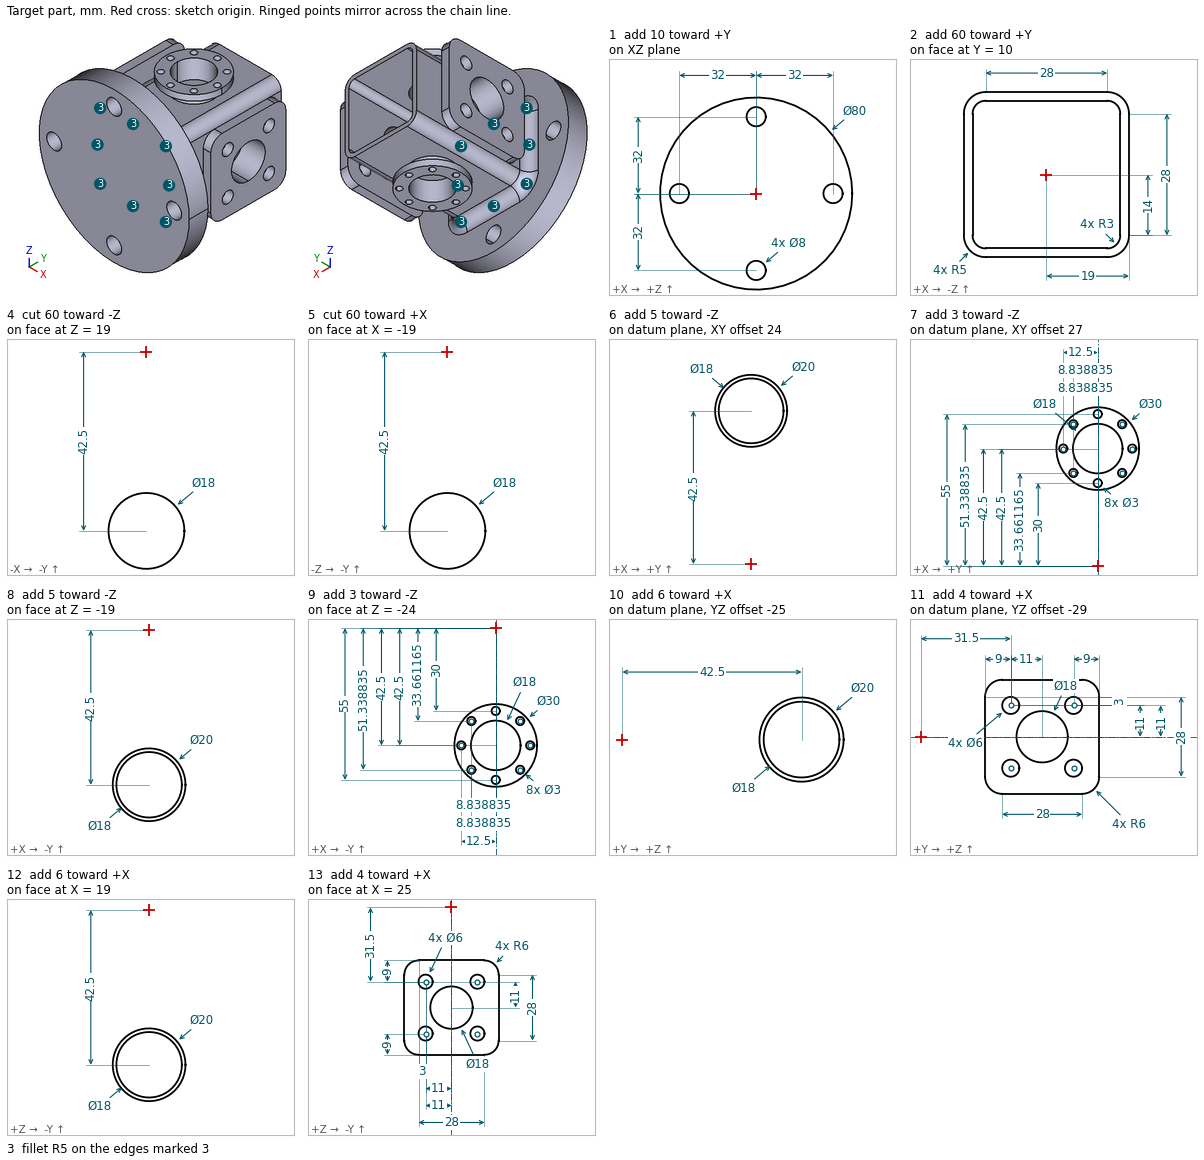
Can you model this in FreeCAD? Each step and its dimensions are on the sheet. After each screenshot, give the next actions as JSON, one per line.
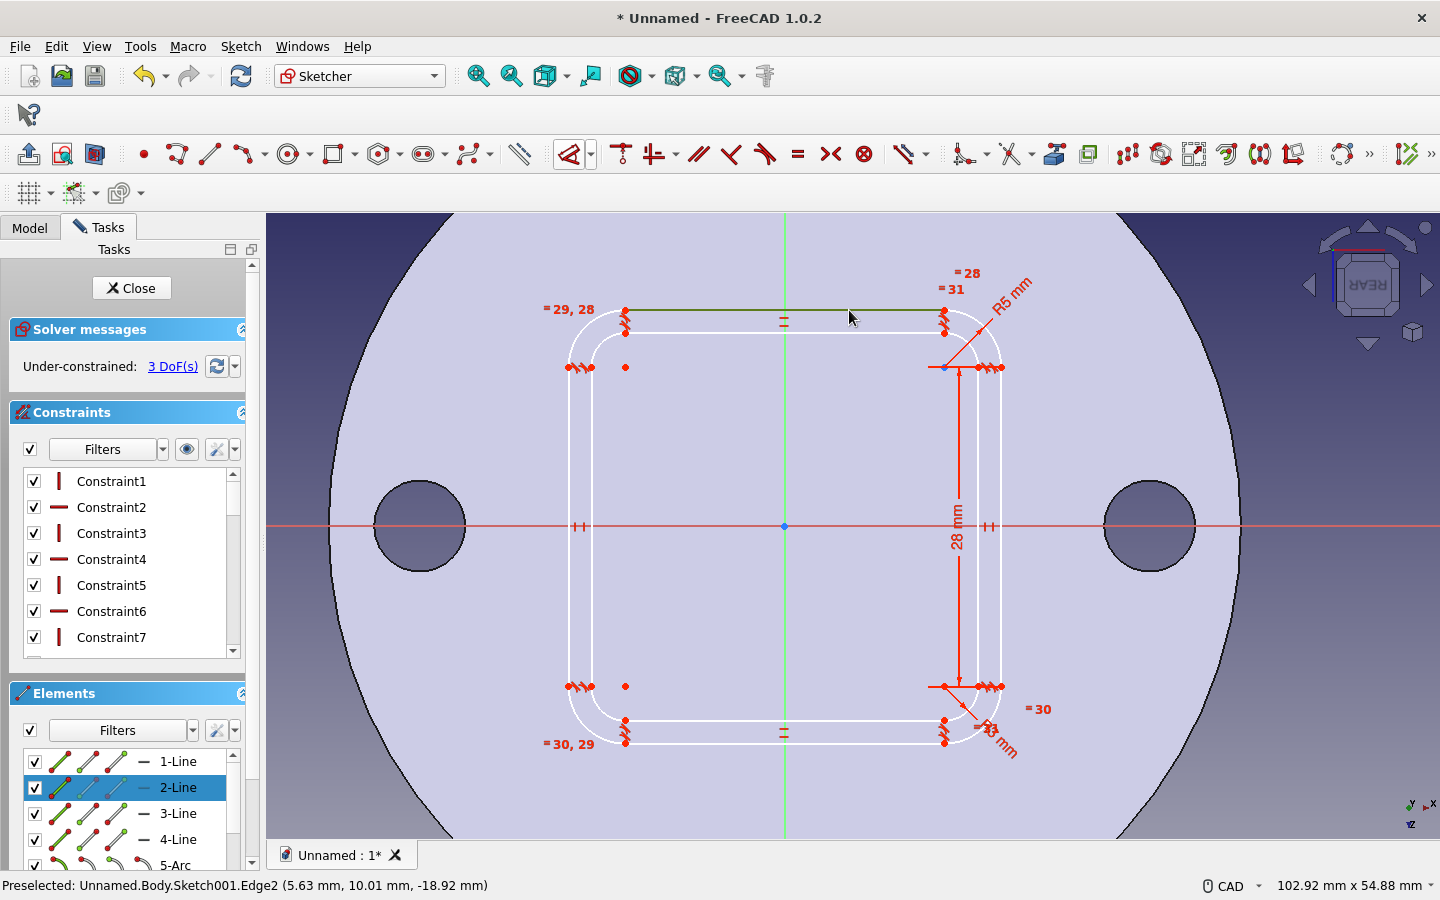
{"action": "key", "text": "l"}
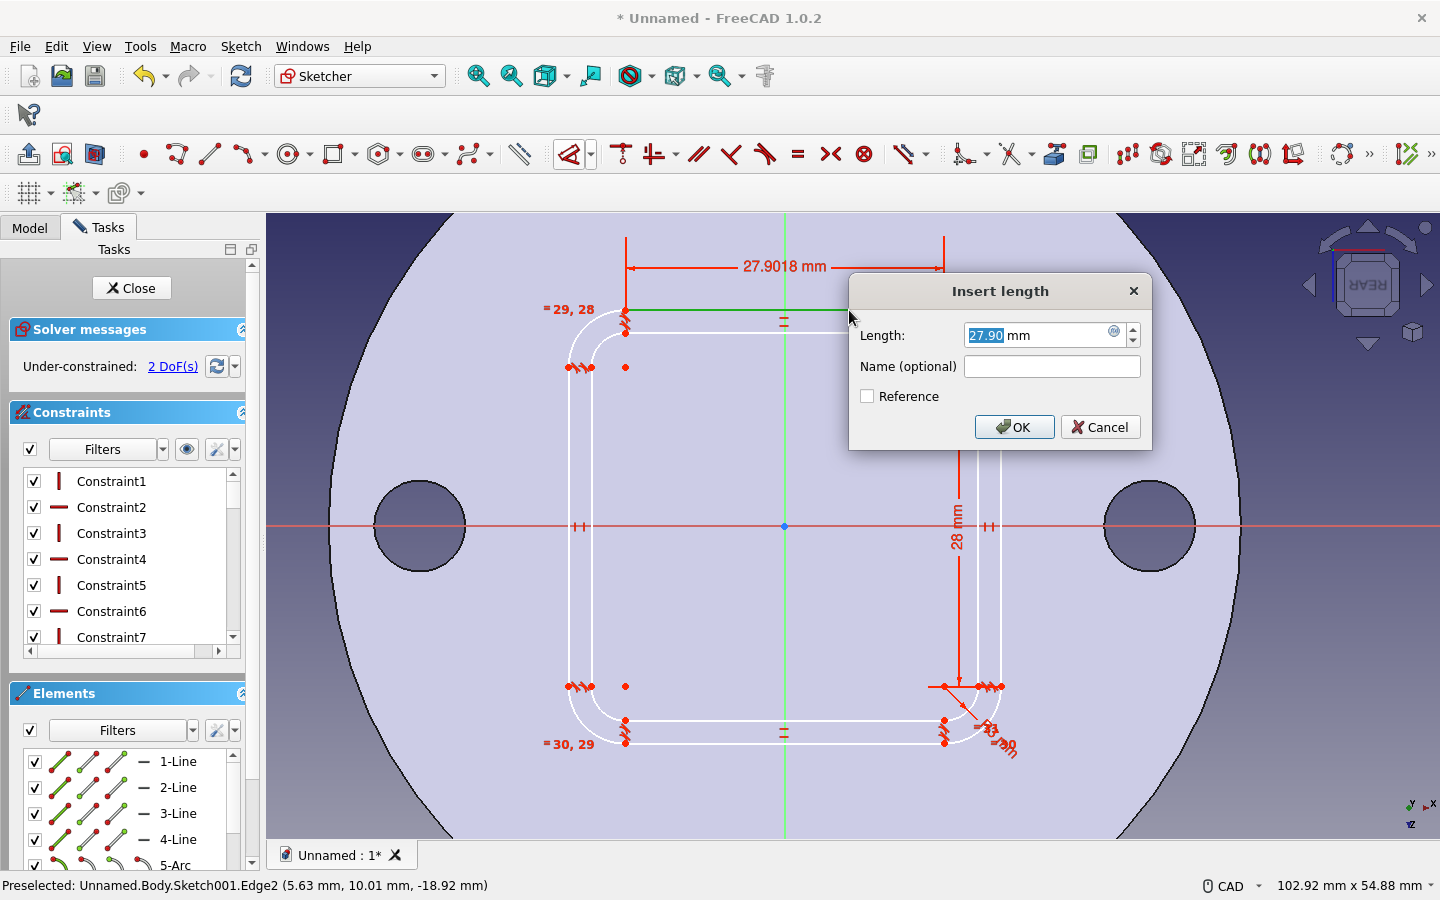
{"action": "type", "text": "28"}
{"action": "key", "text": "Return"}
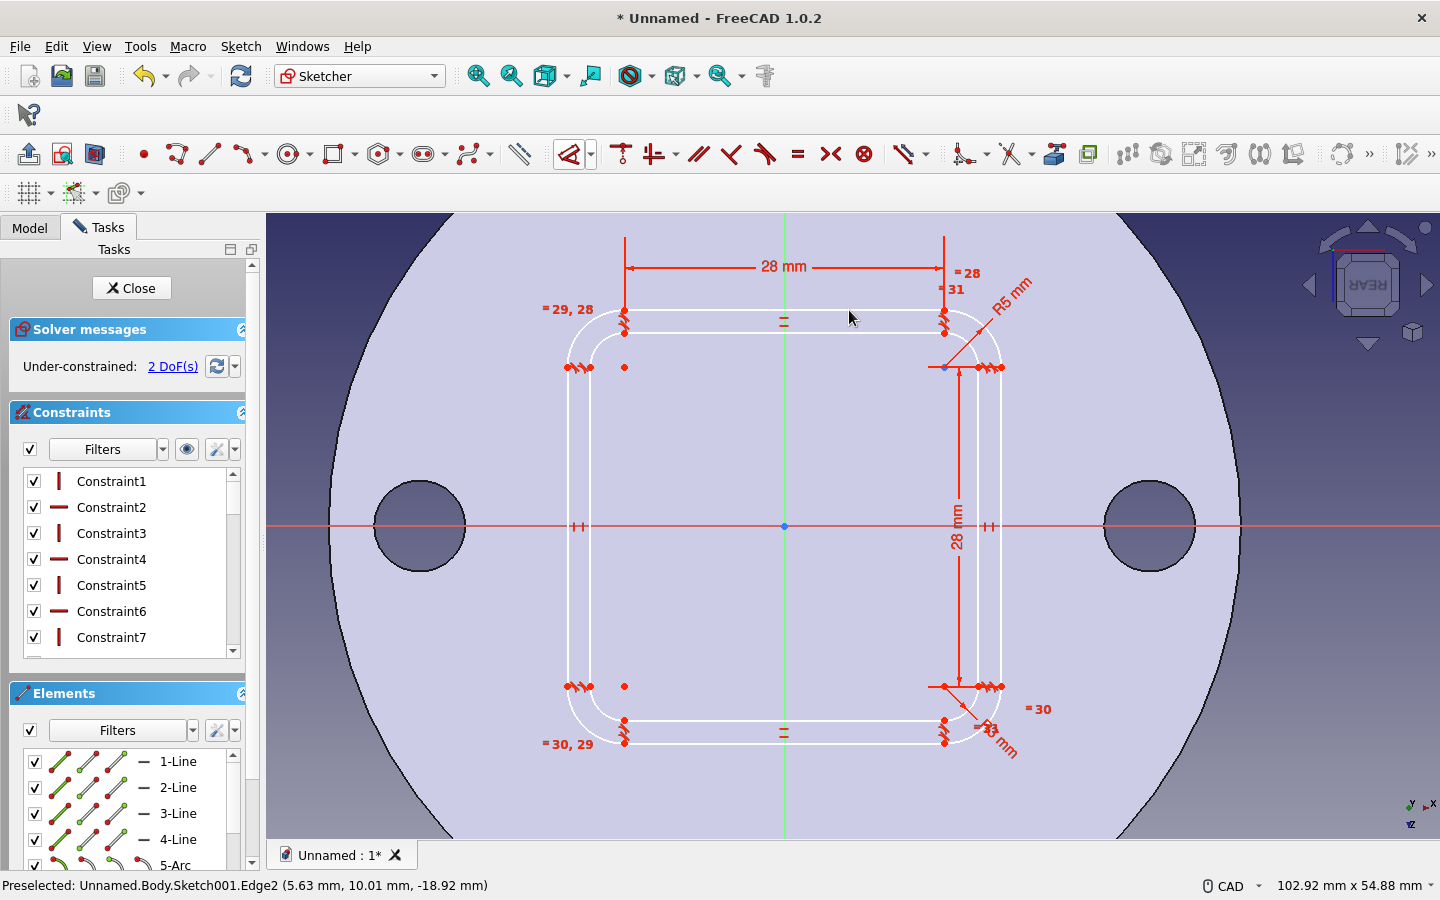
{"action": "left_click", "coordinate": [1001, 687]}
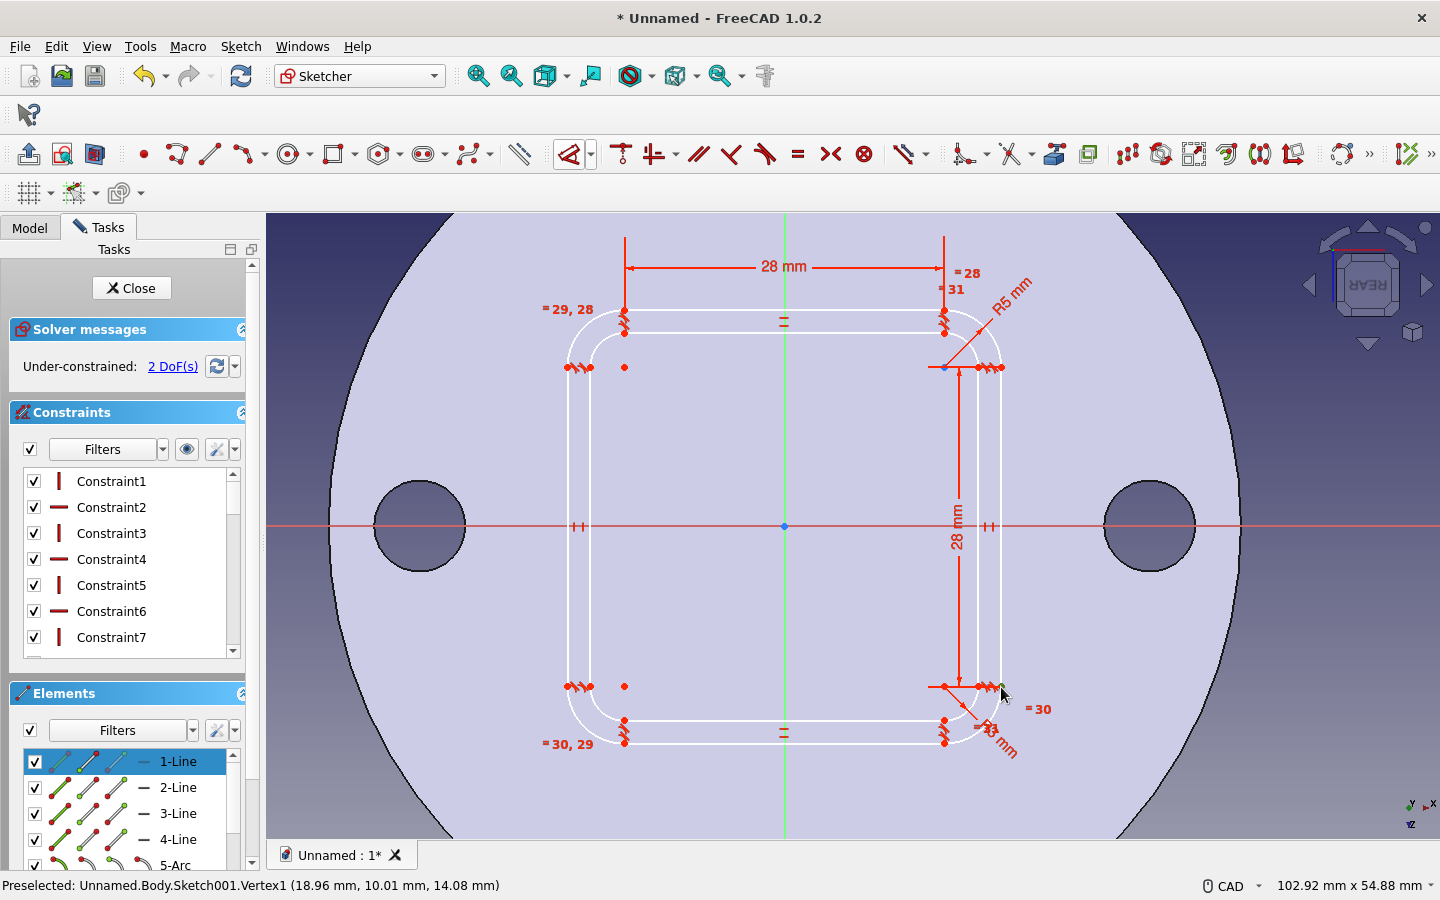
{"action": "key", "text": "l"}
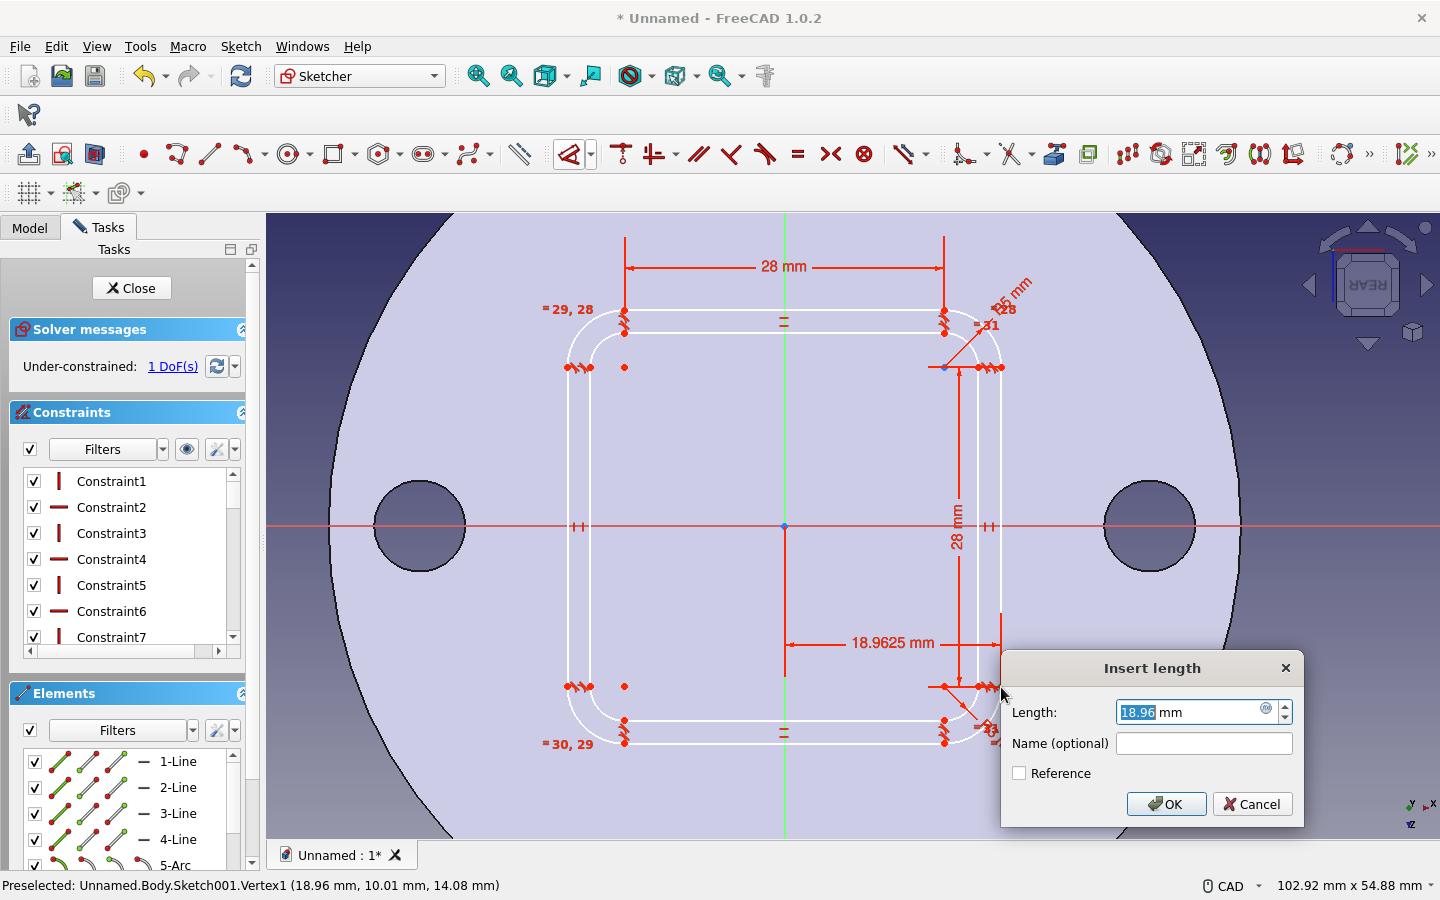
{"action": "type", "text": "19"}
{"action": "key", "text": "Return"}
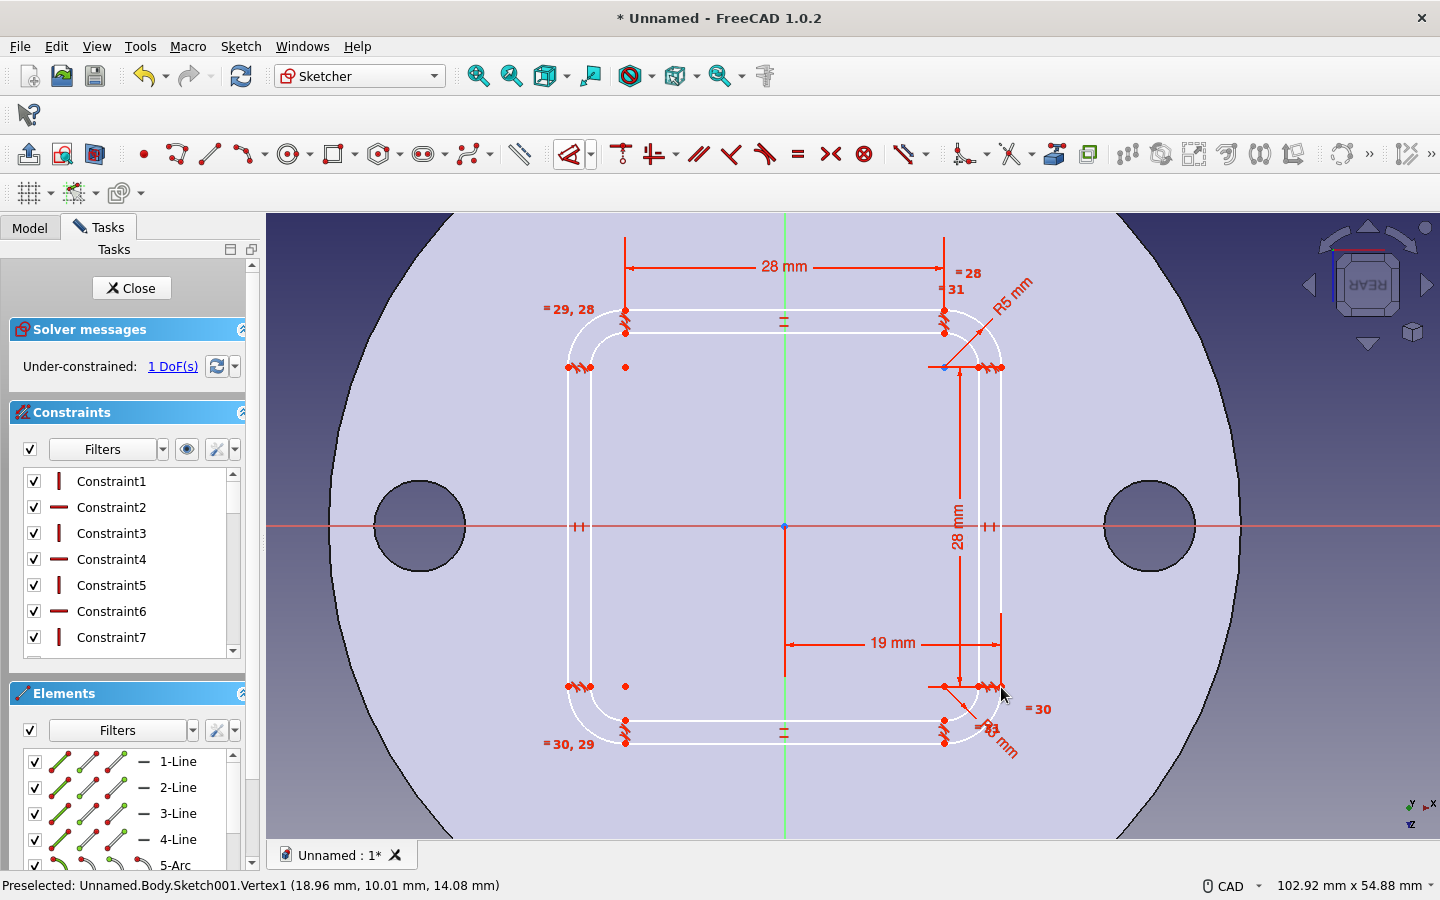
{"action": "left_click", "coordinate": [1001, 687]}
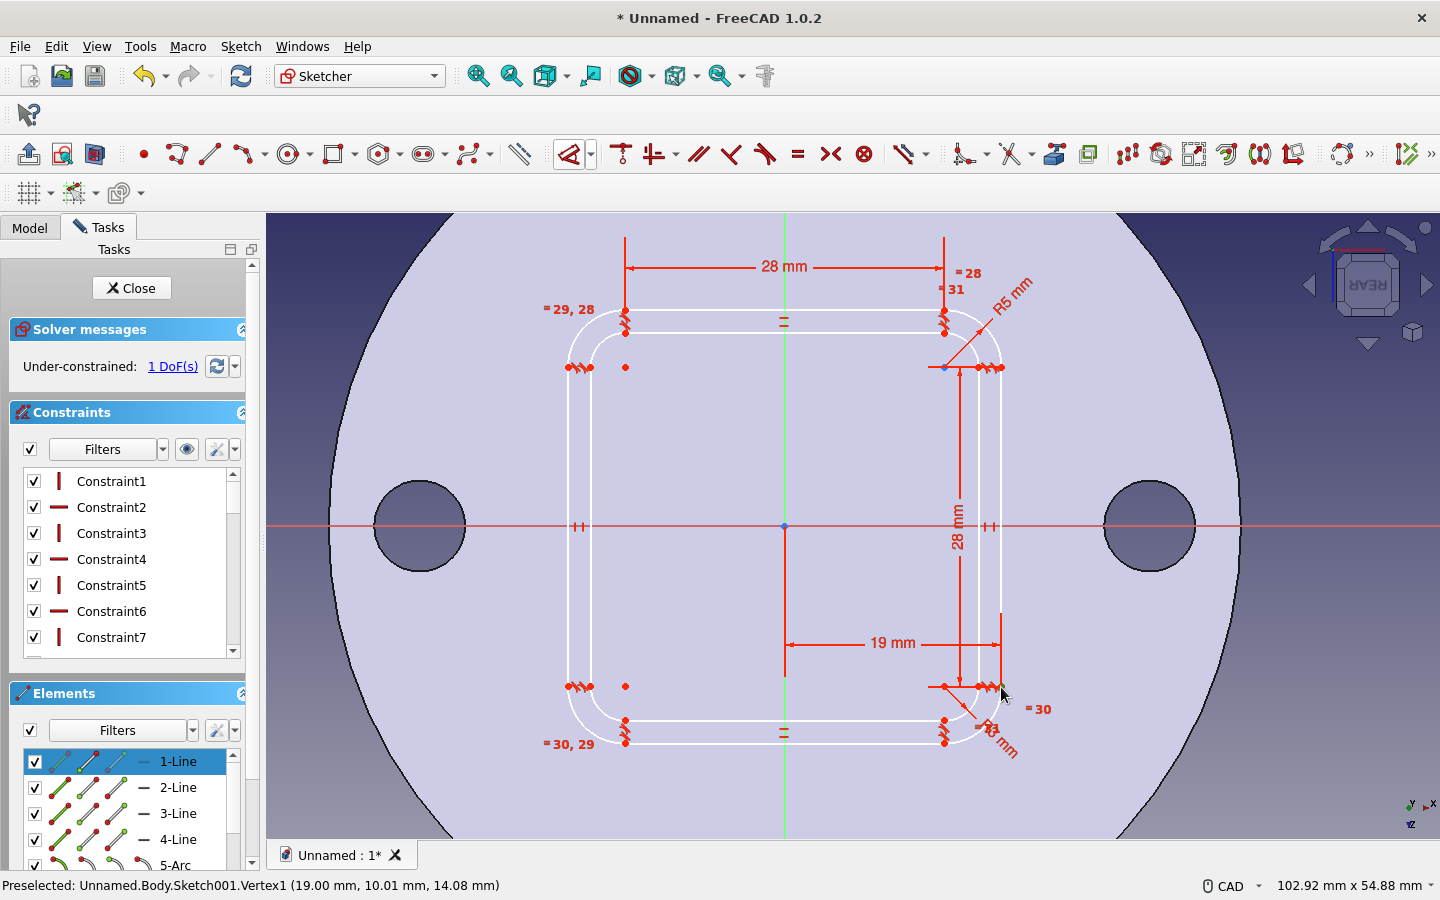
{"action": "key", "text": "i"}